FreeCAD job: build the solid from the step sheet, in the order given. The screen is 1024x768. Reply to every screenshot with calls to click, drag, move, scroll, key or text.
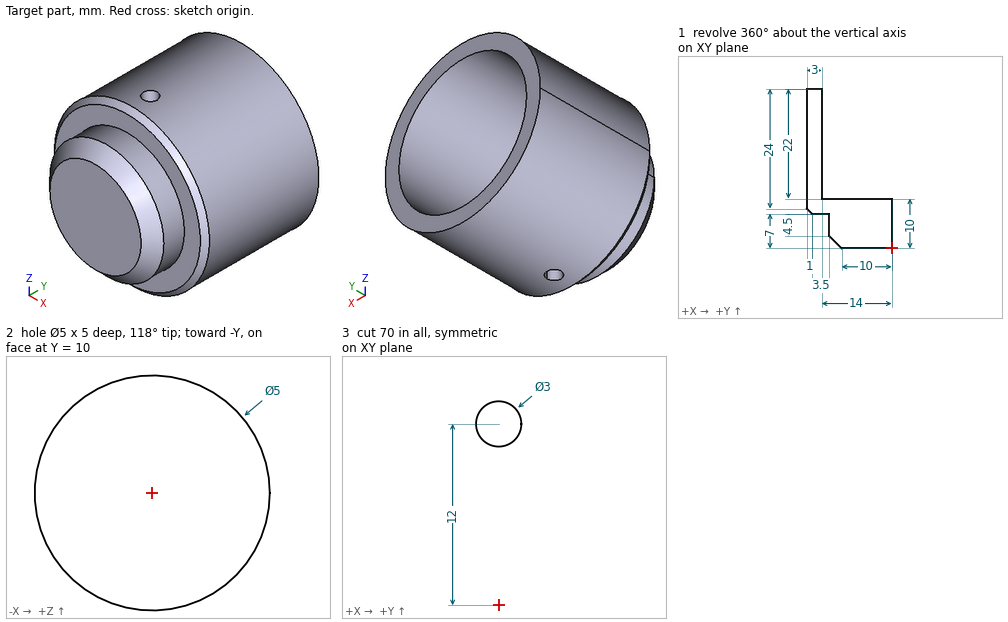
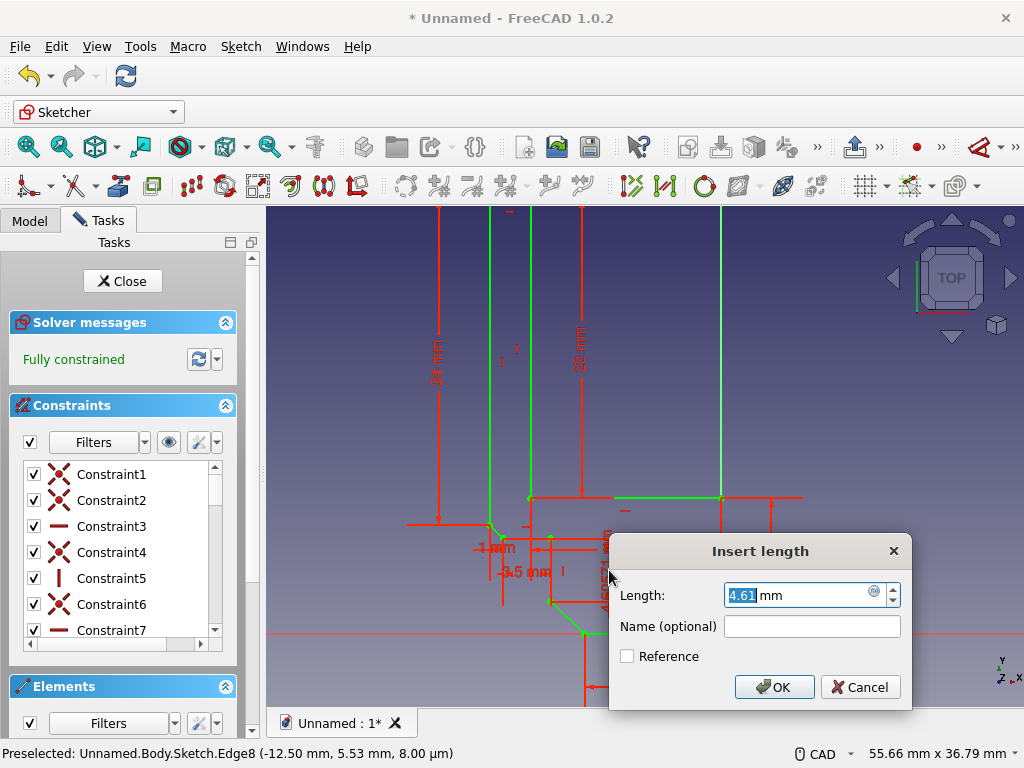
text(4.5)
key(Return)
key(Escape)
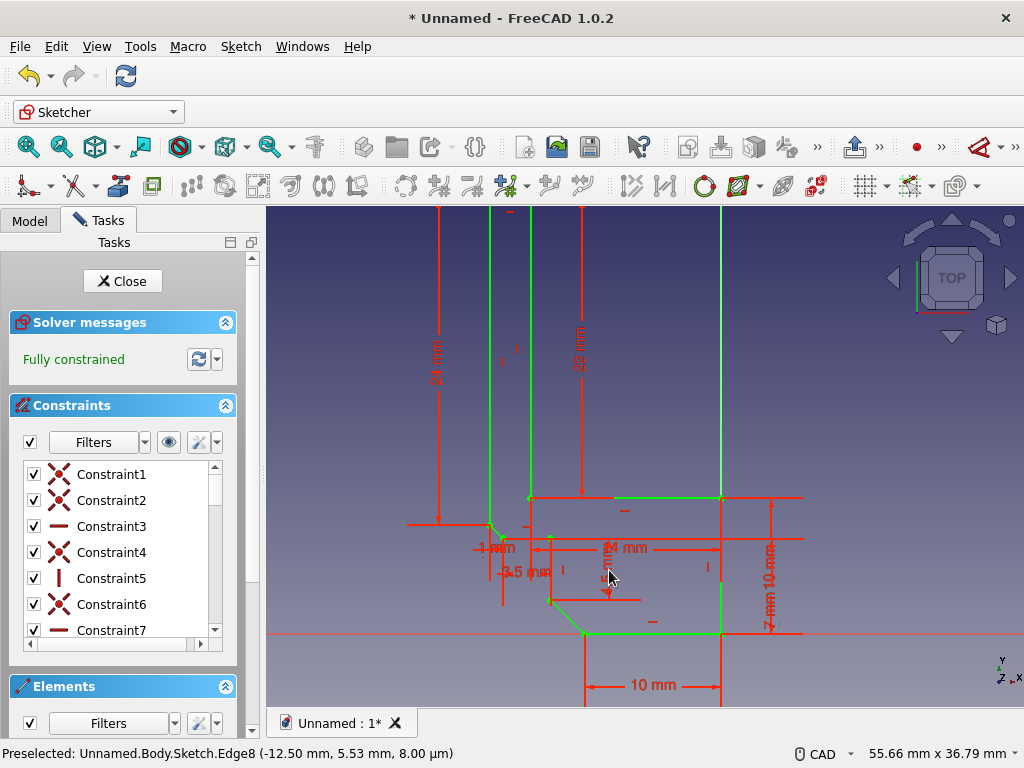
click(123, 281)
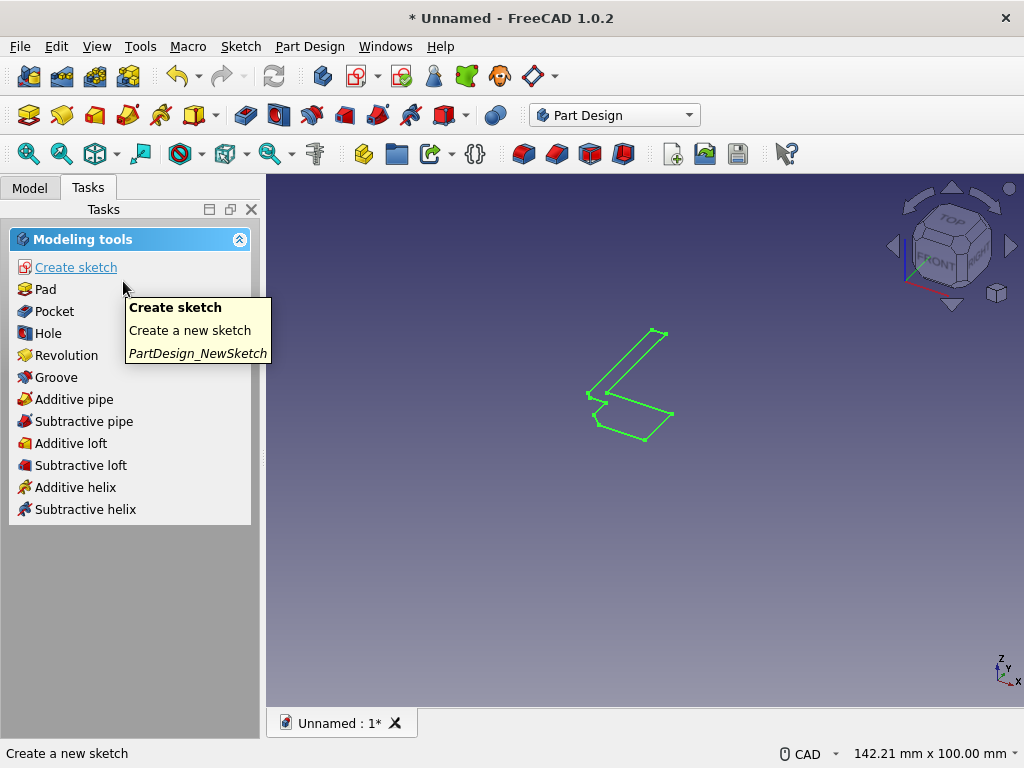
click(62, 116)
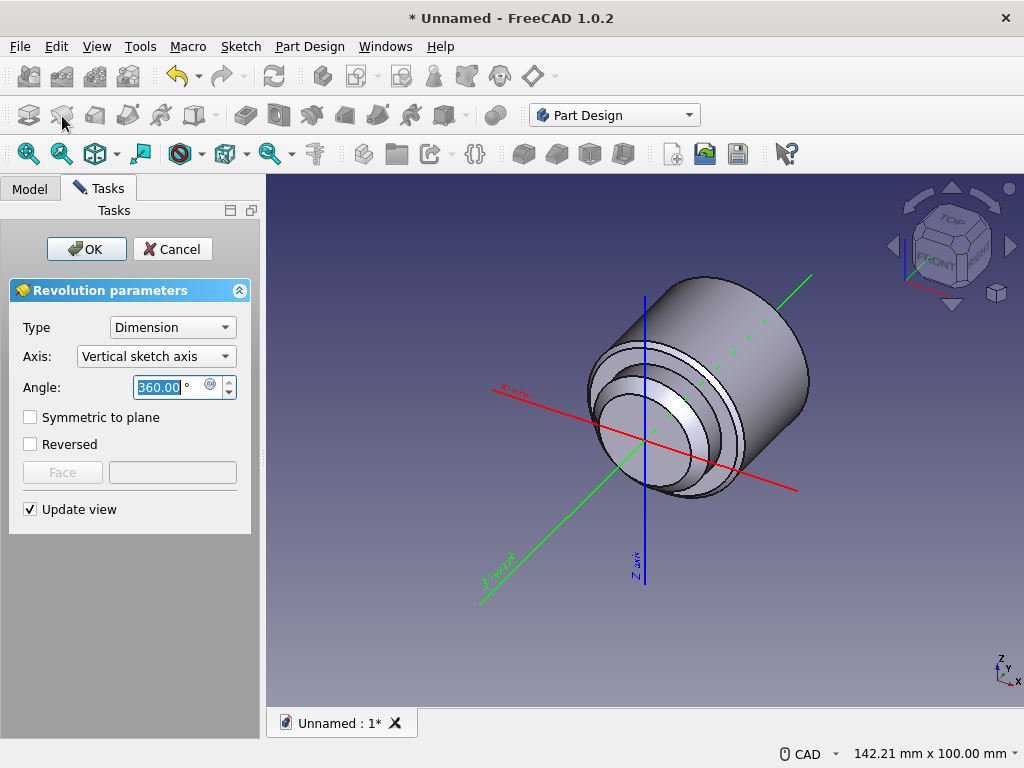
click(87, 249)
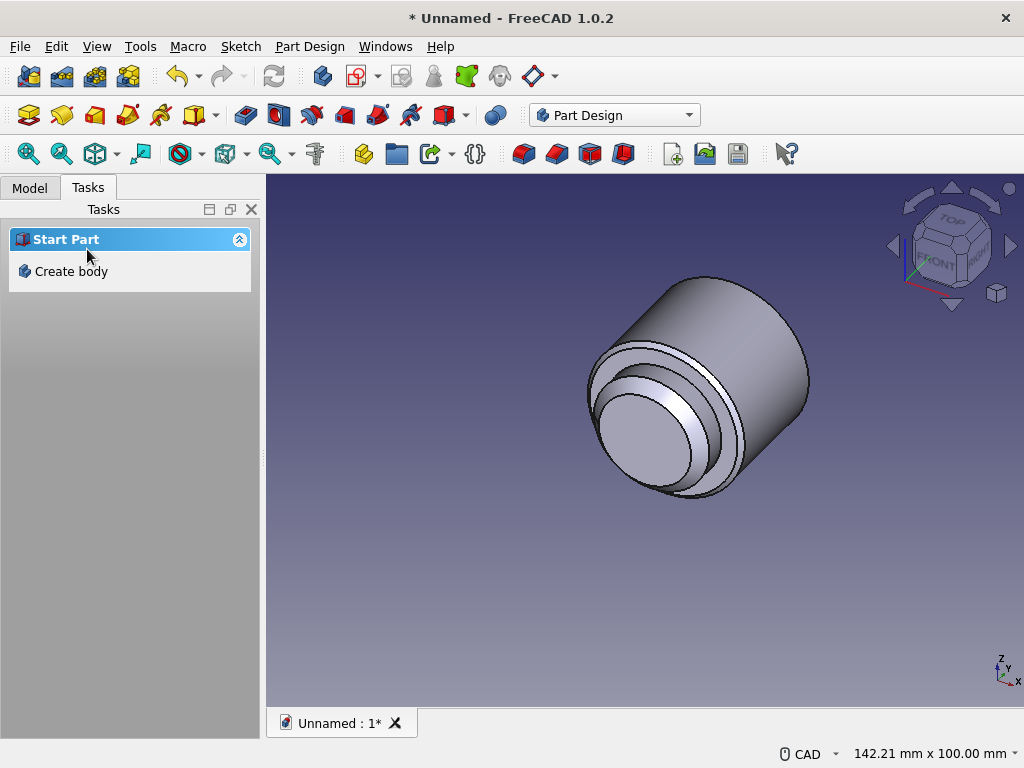
key(4)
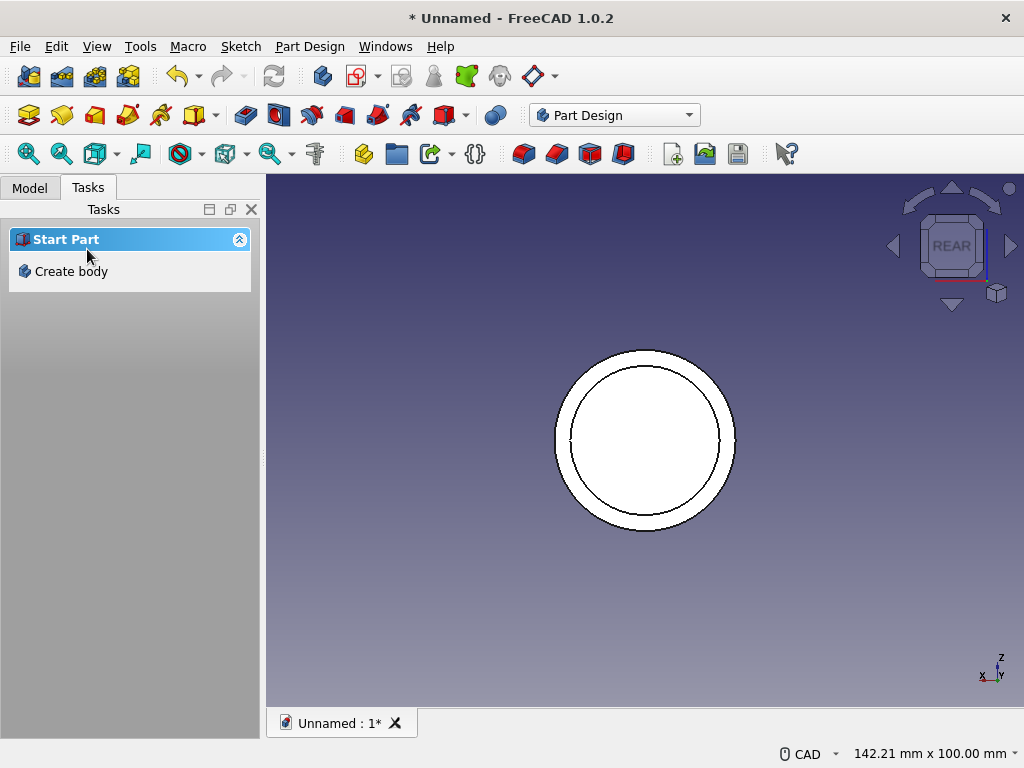
key(v)
key(f)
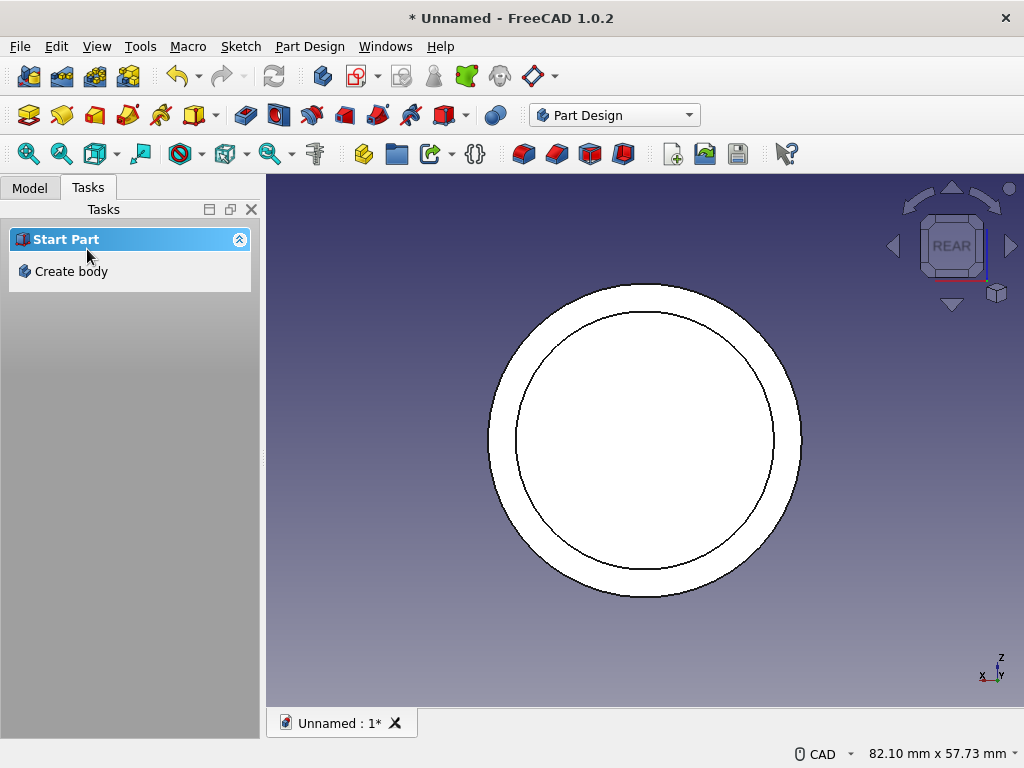
click(645, 440)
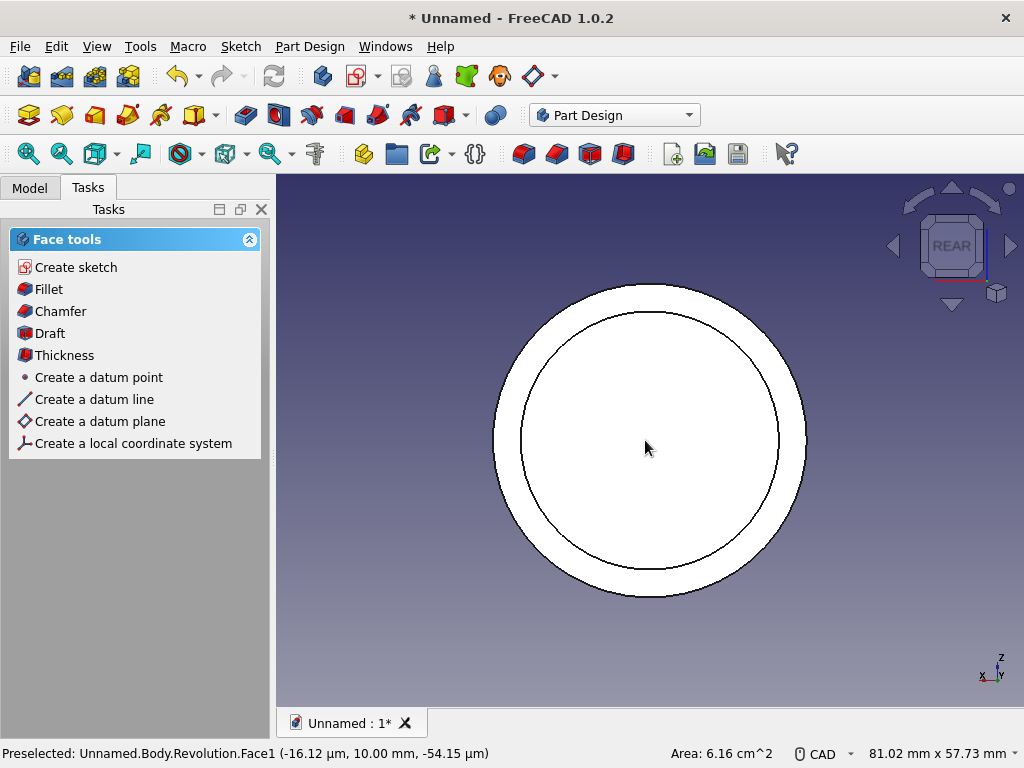
click(356, 76)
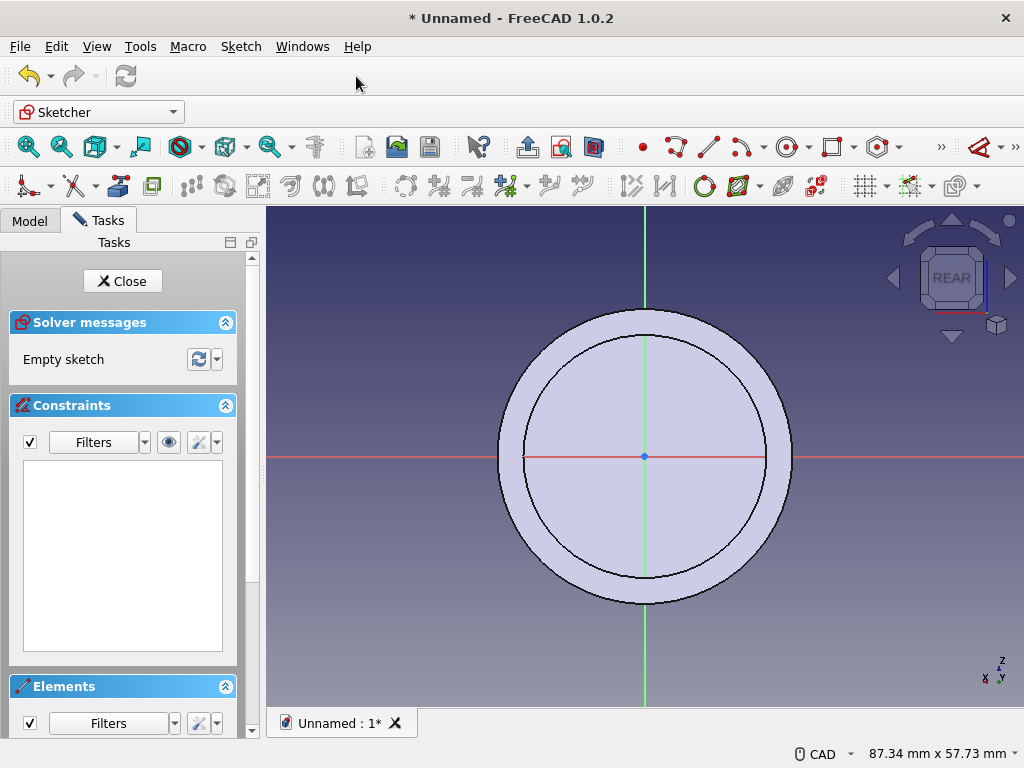
click(594, 148)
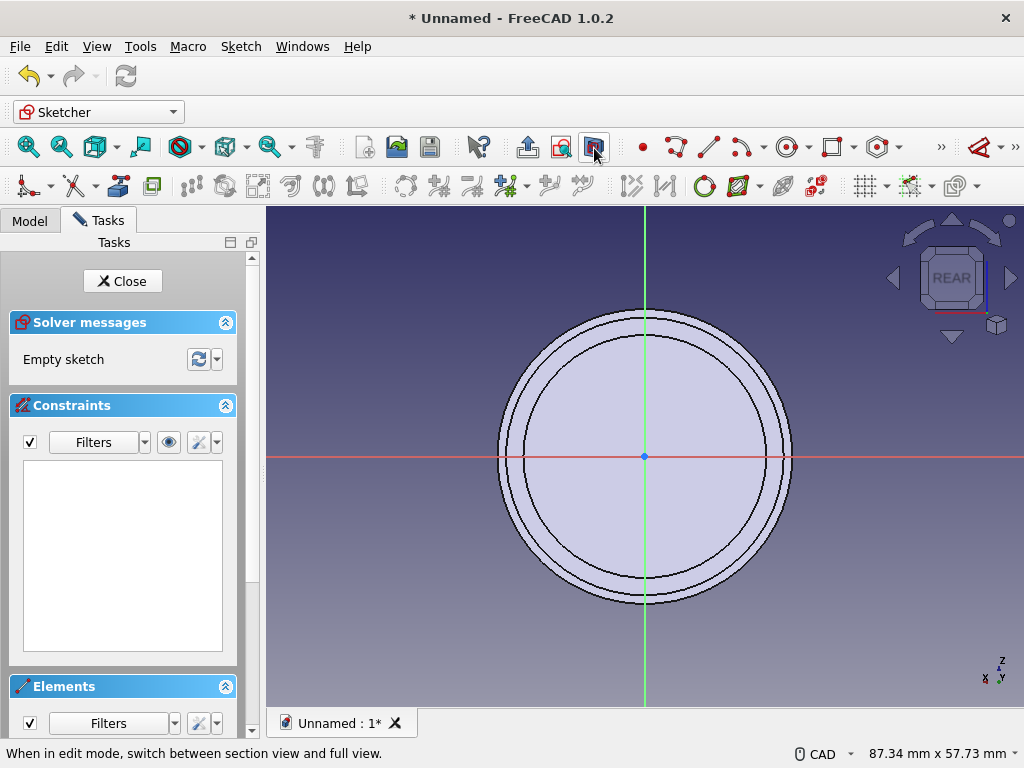
scroll(656, 456, up, 10)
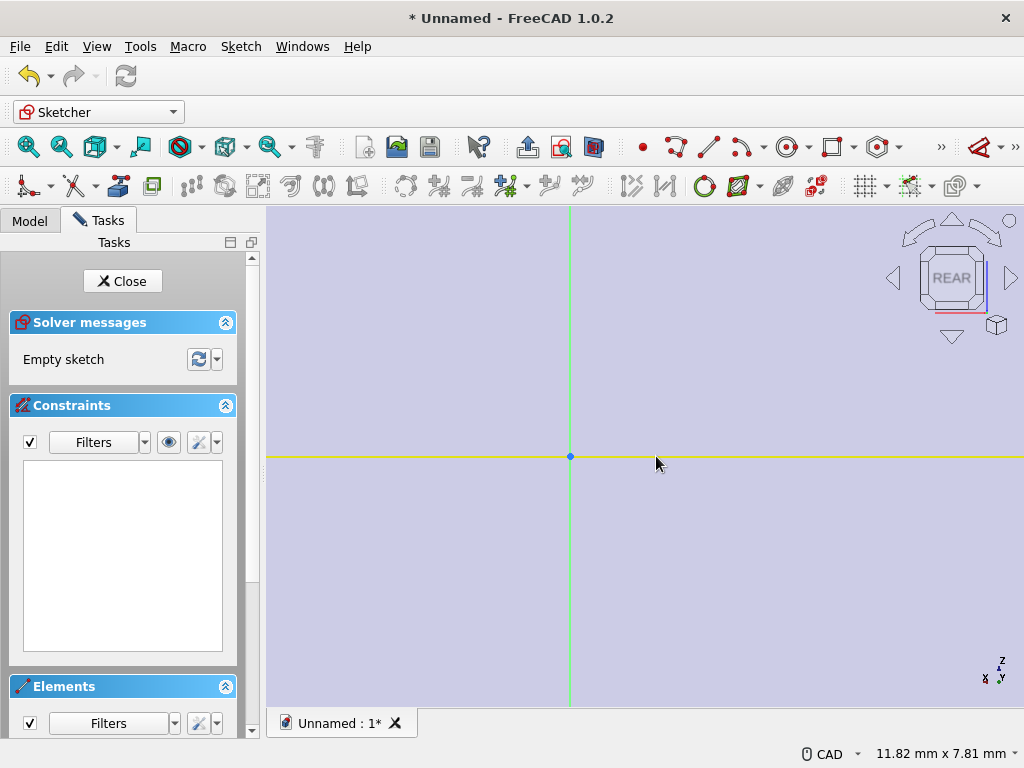
click(786, 148)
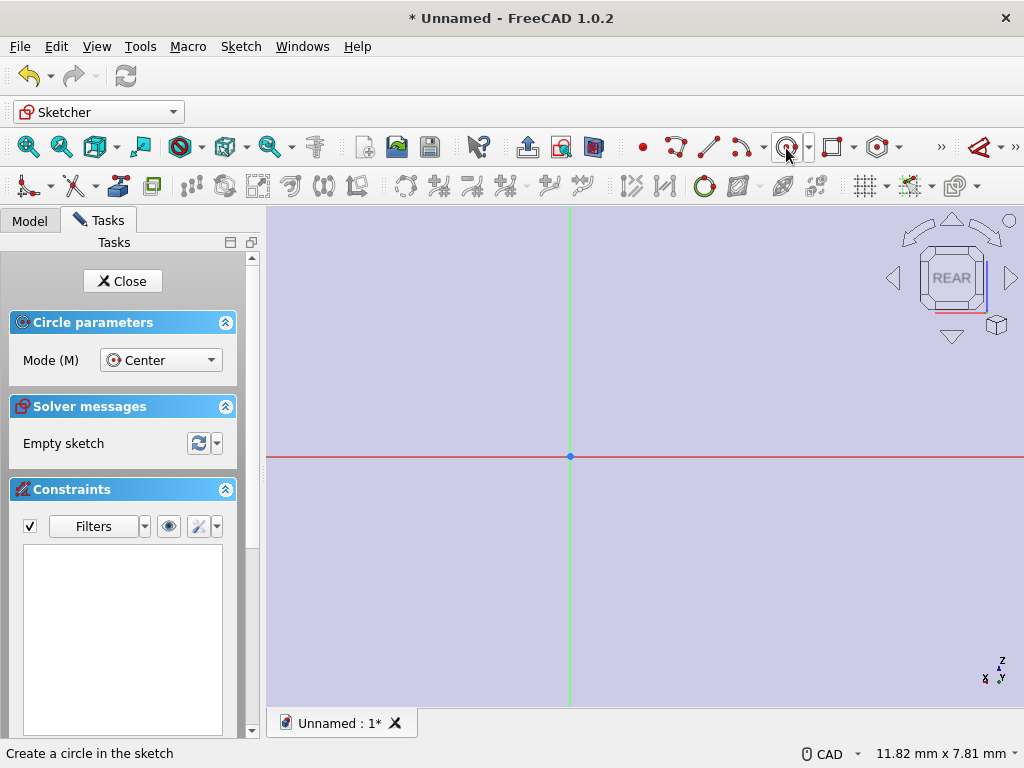
click(570, 456)
click(684, 343)
key(Escape)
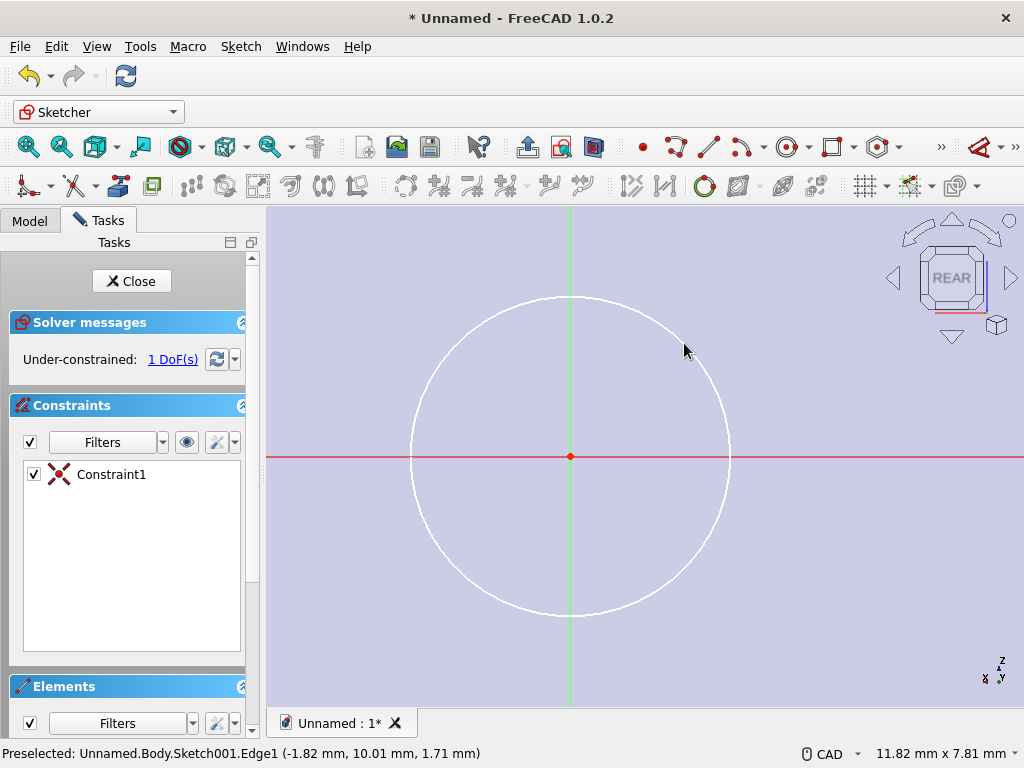
key(d)